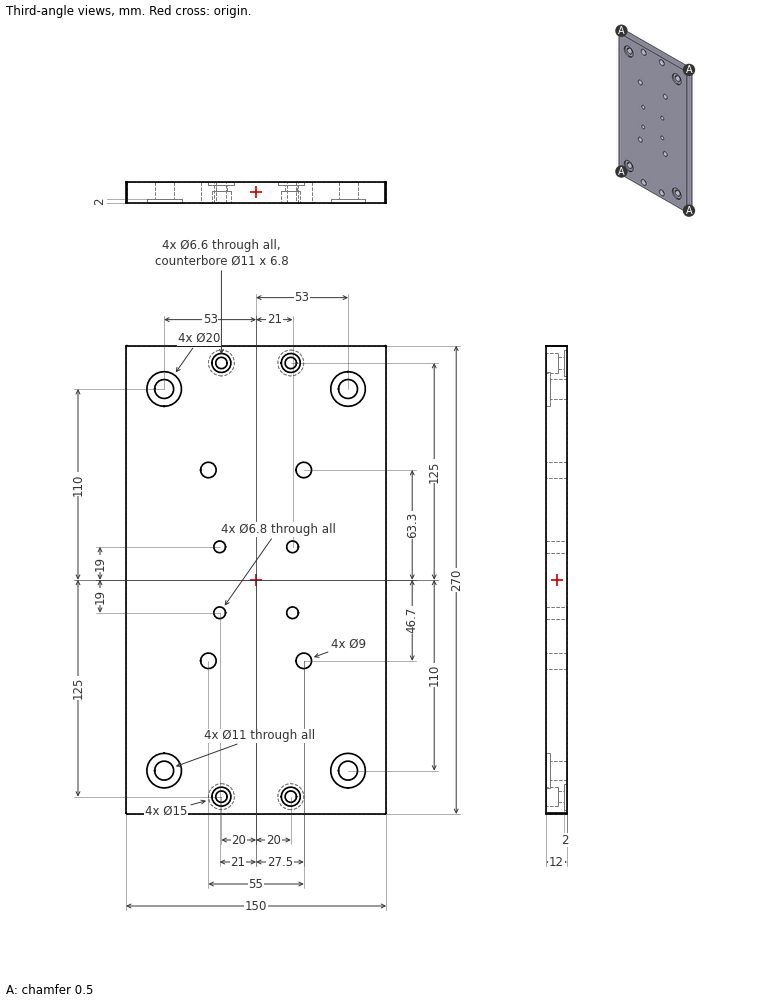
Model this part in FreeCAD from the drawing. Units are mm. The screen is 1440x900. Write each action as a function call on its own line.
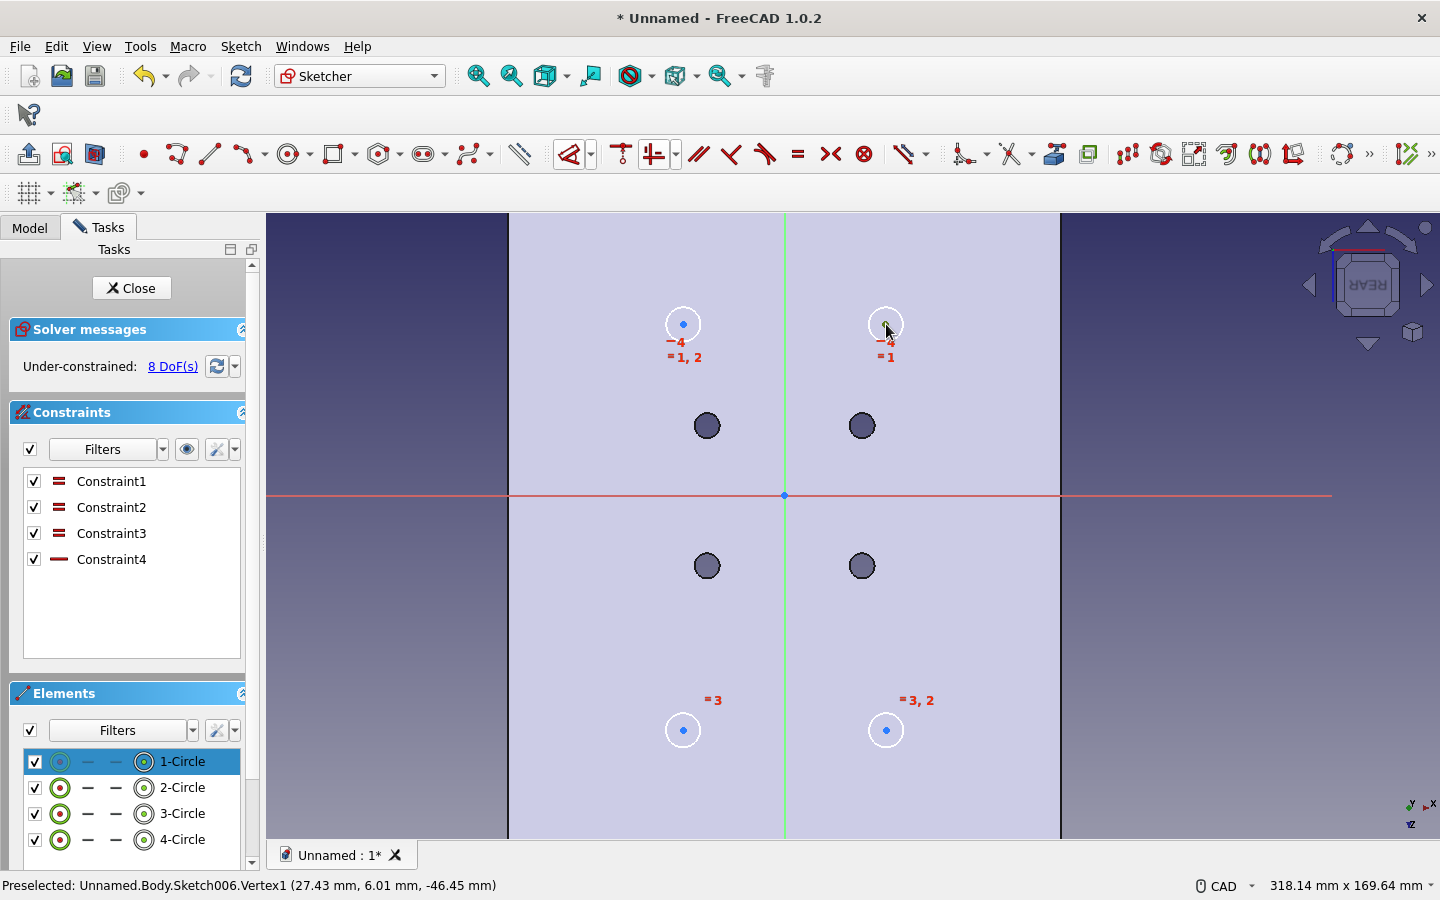
click(886, 730)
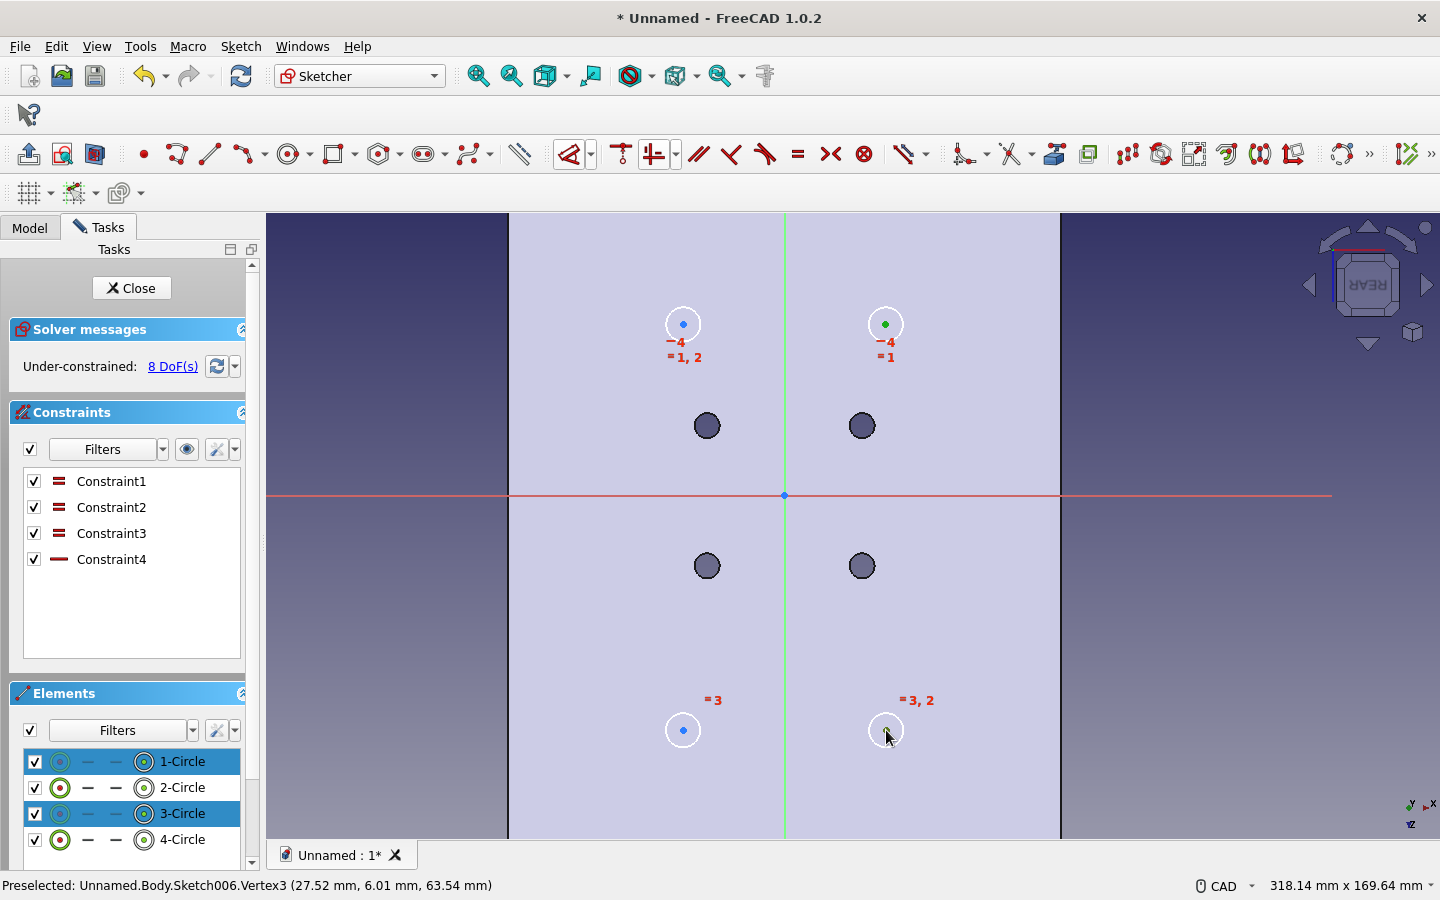
key(v)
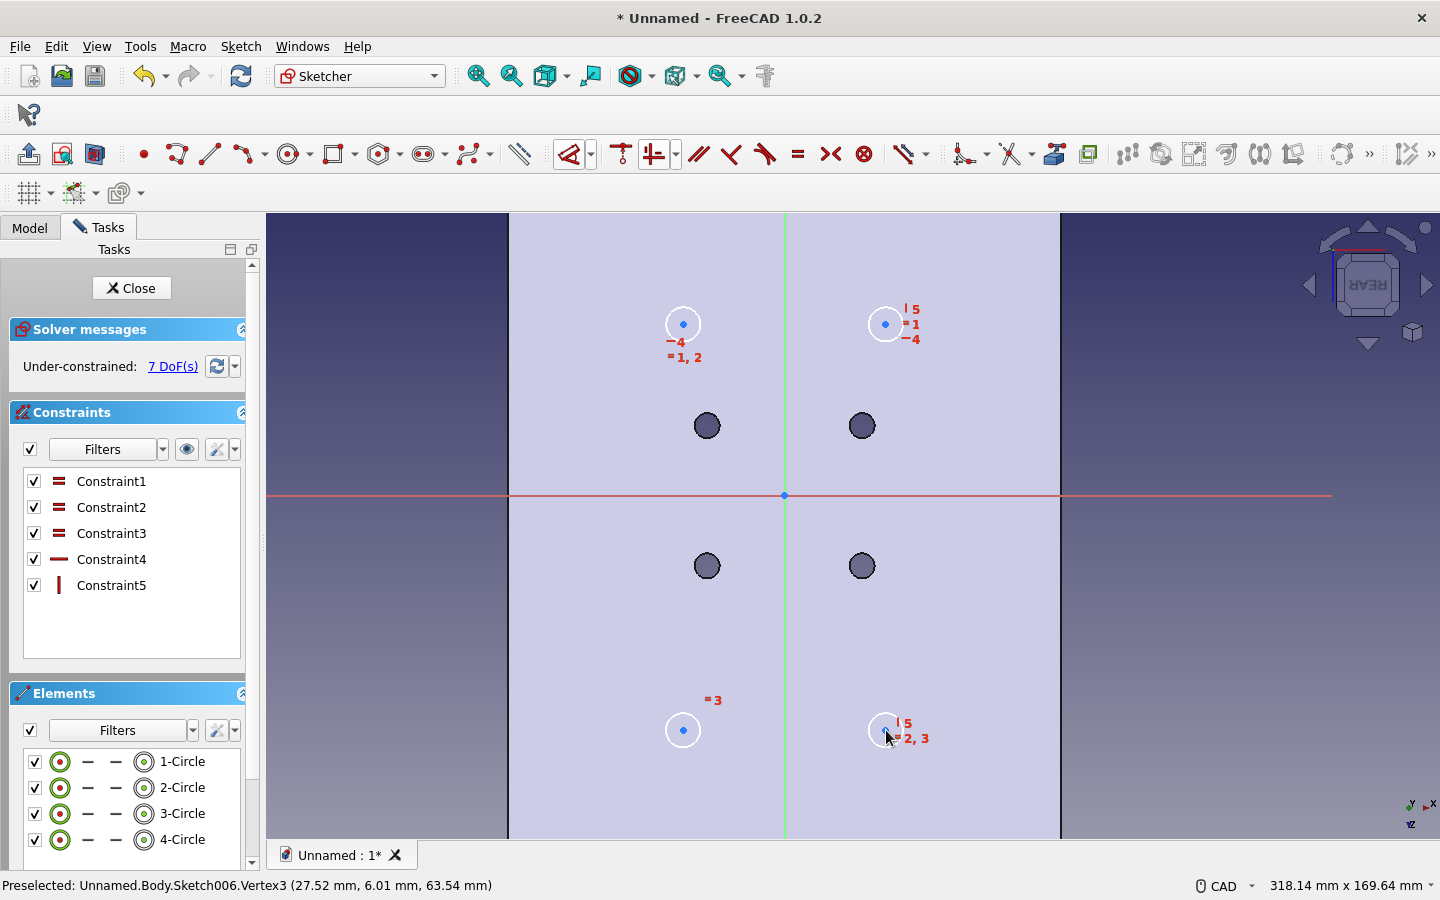
click(683, 324)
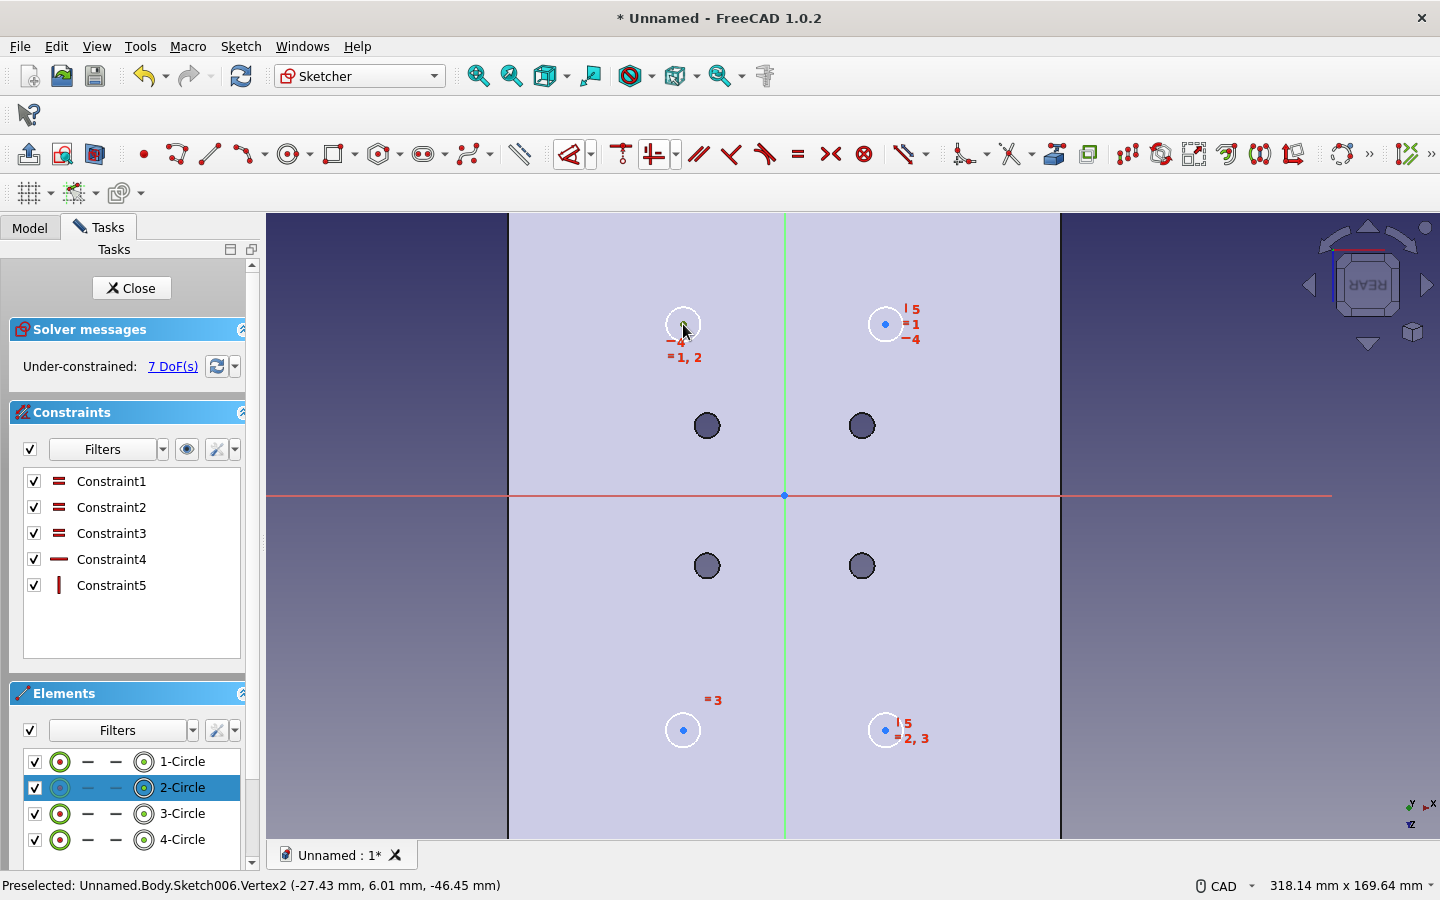
click(683, 730)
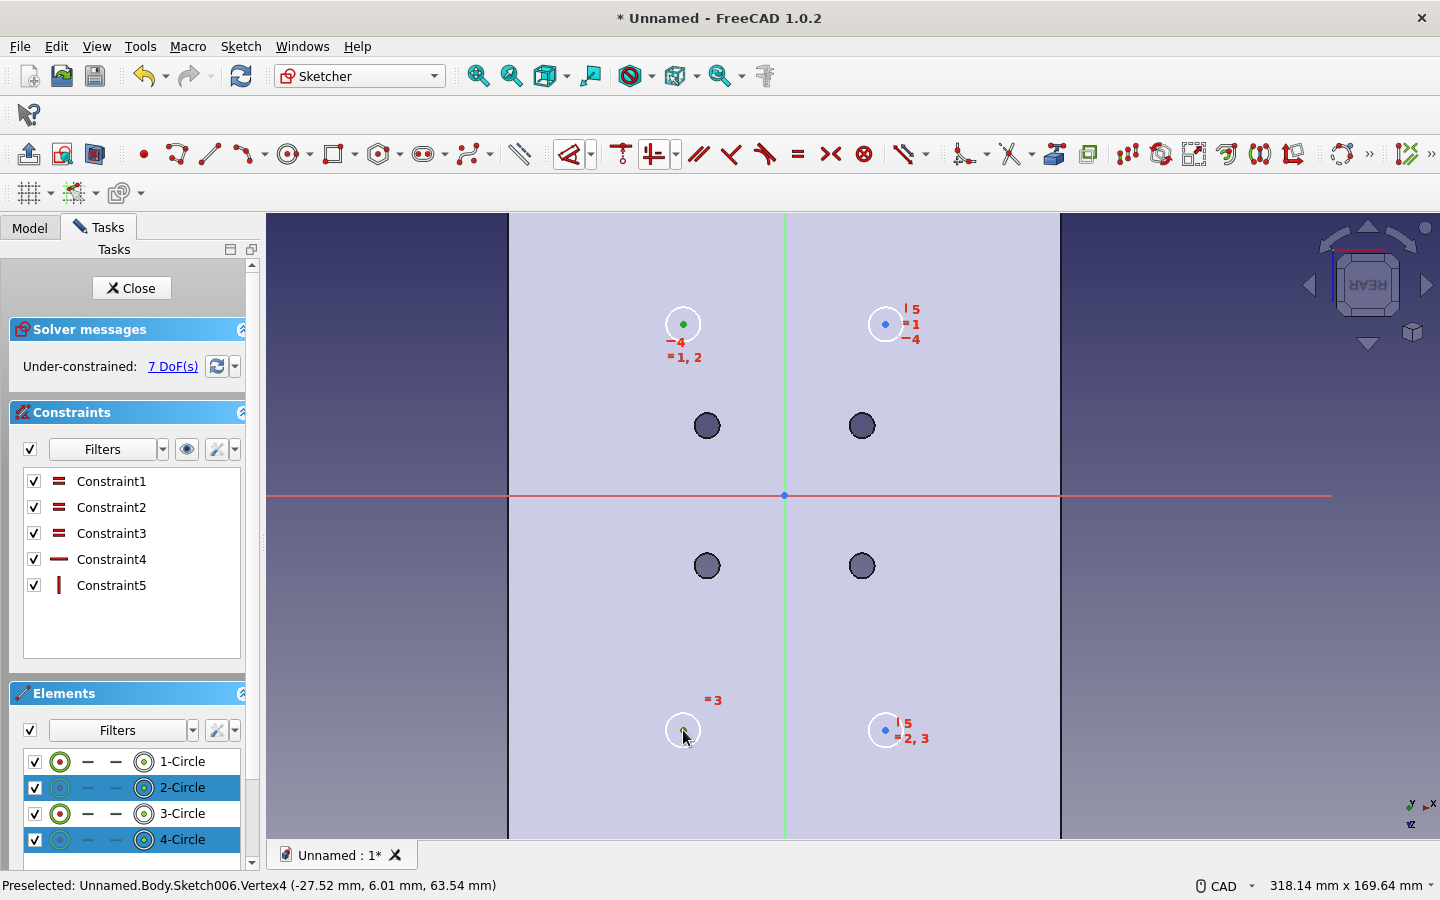
click(676, 154)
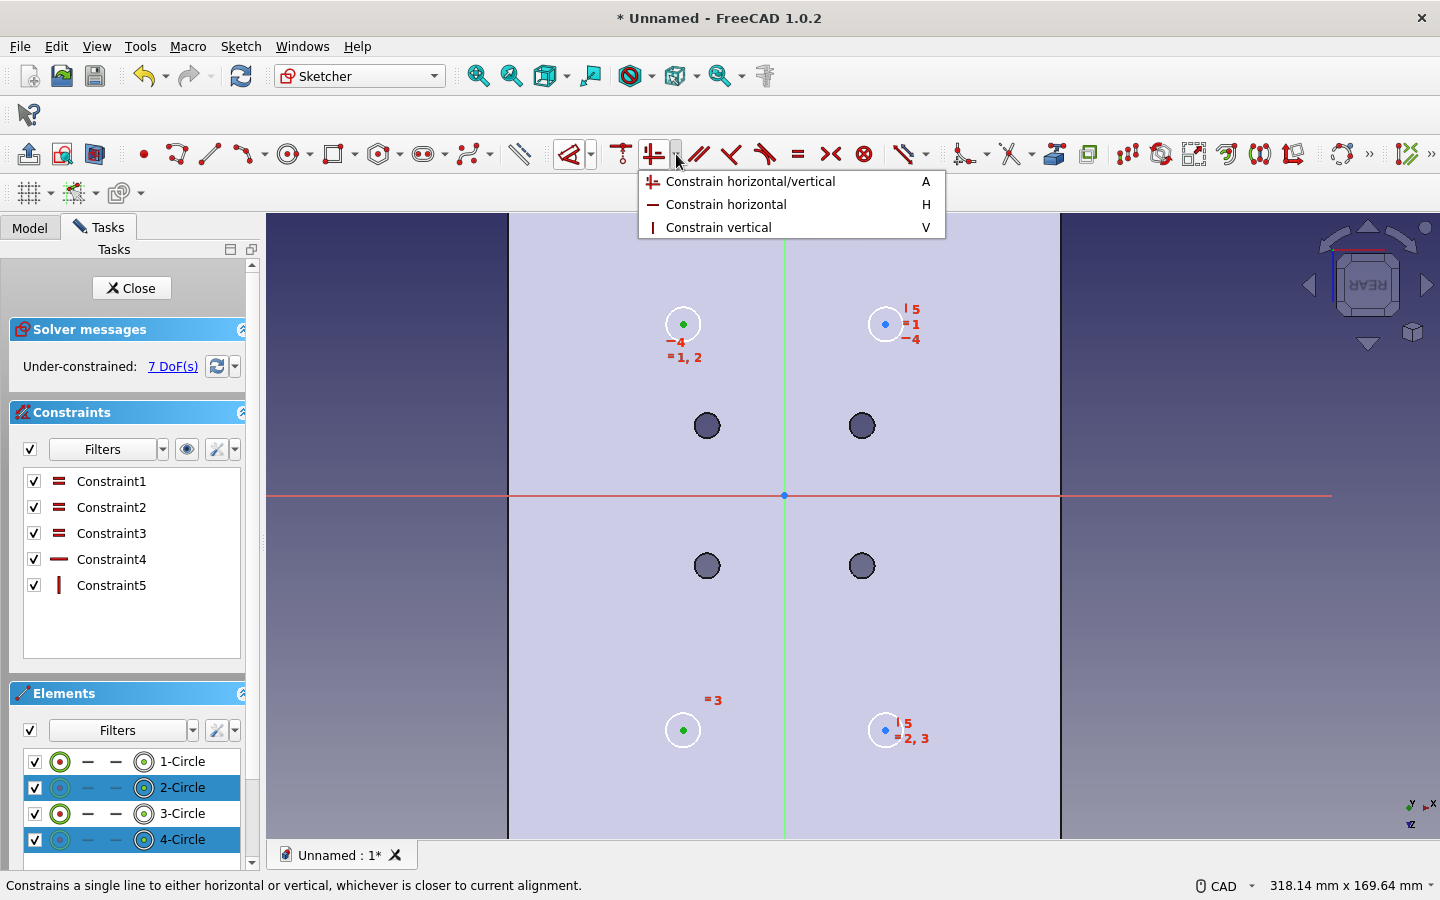
click(792, 228)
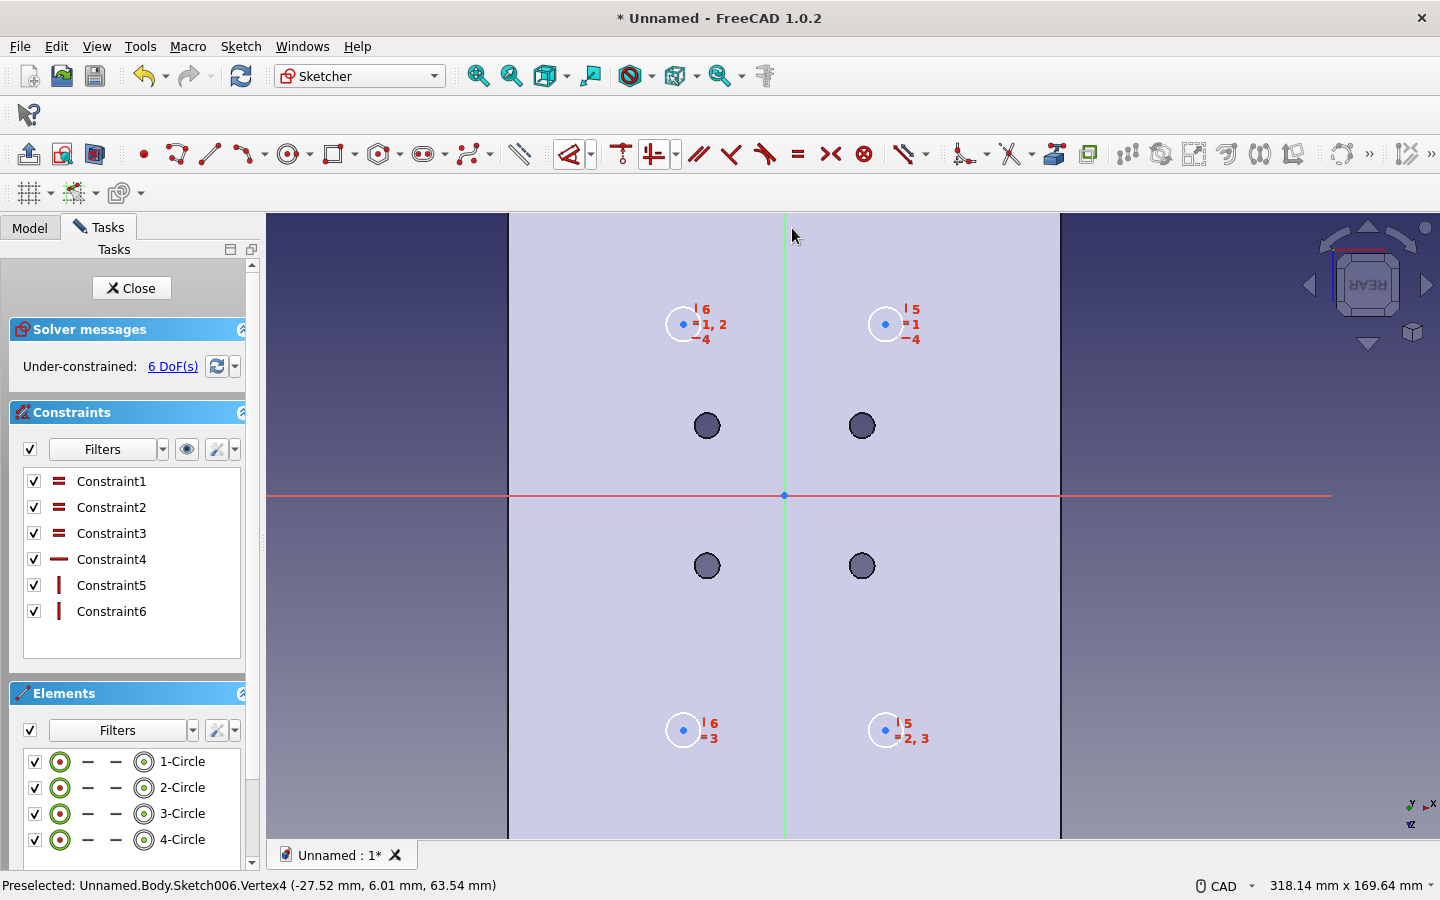
click(886, 730)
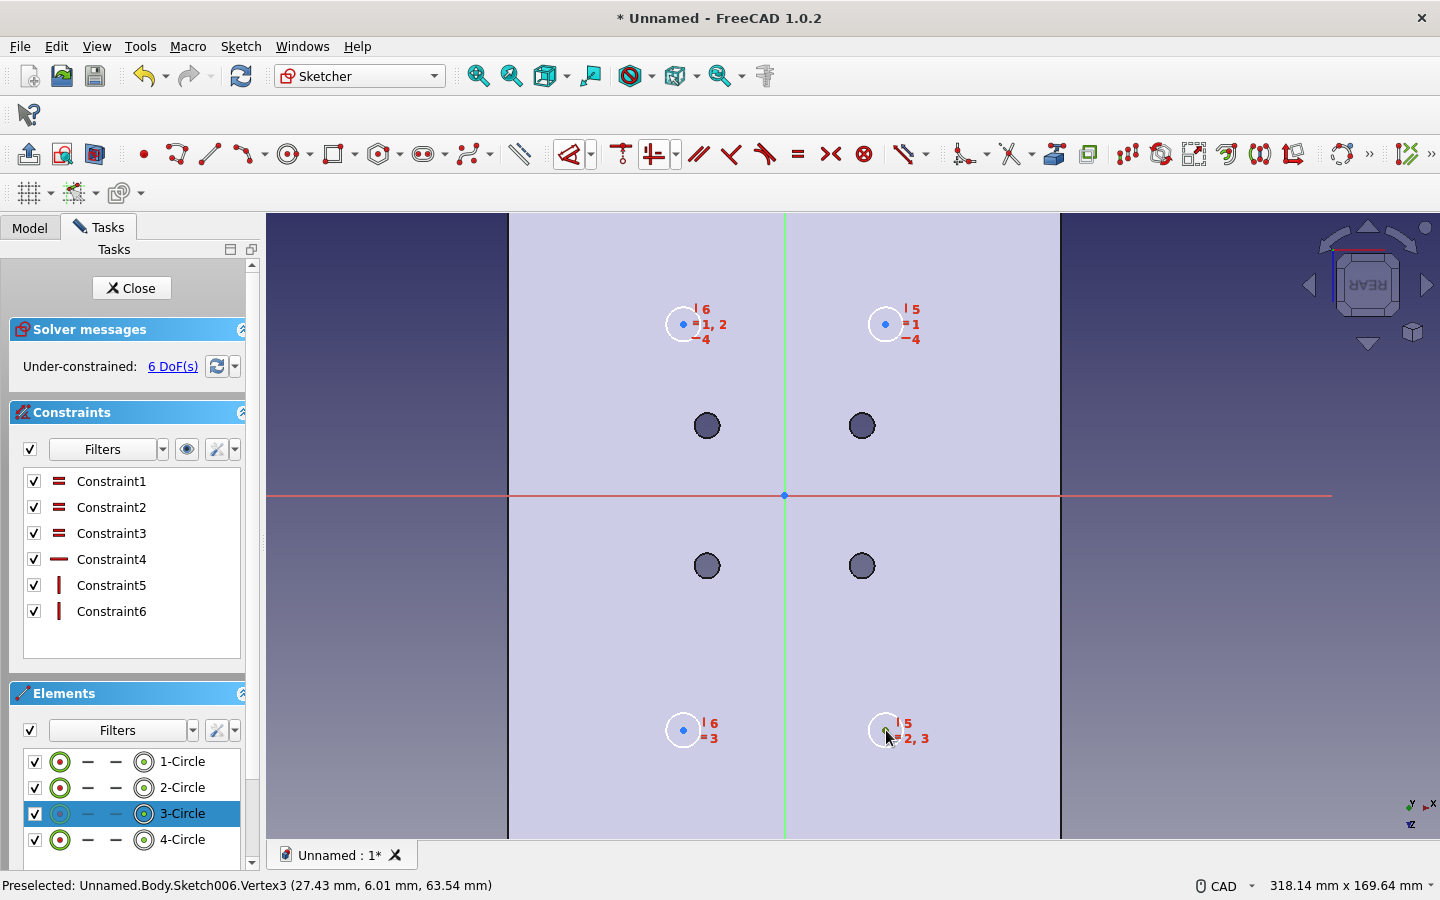
click(683, 730)